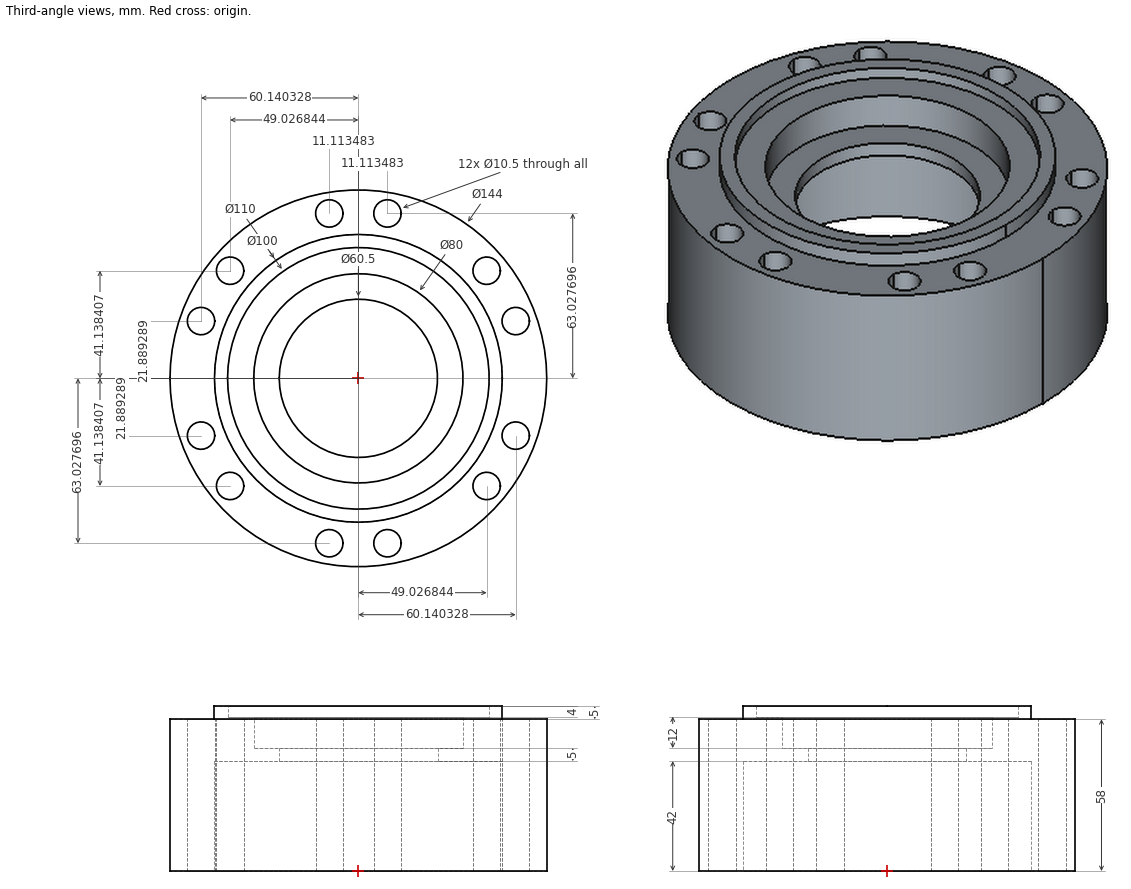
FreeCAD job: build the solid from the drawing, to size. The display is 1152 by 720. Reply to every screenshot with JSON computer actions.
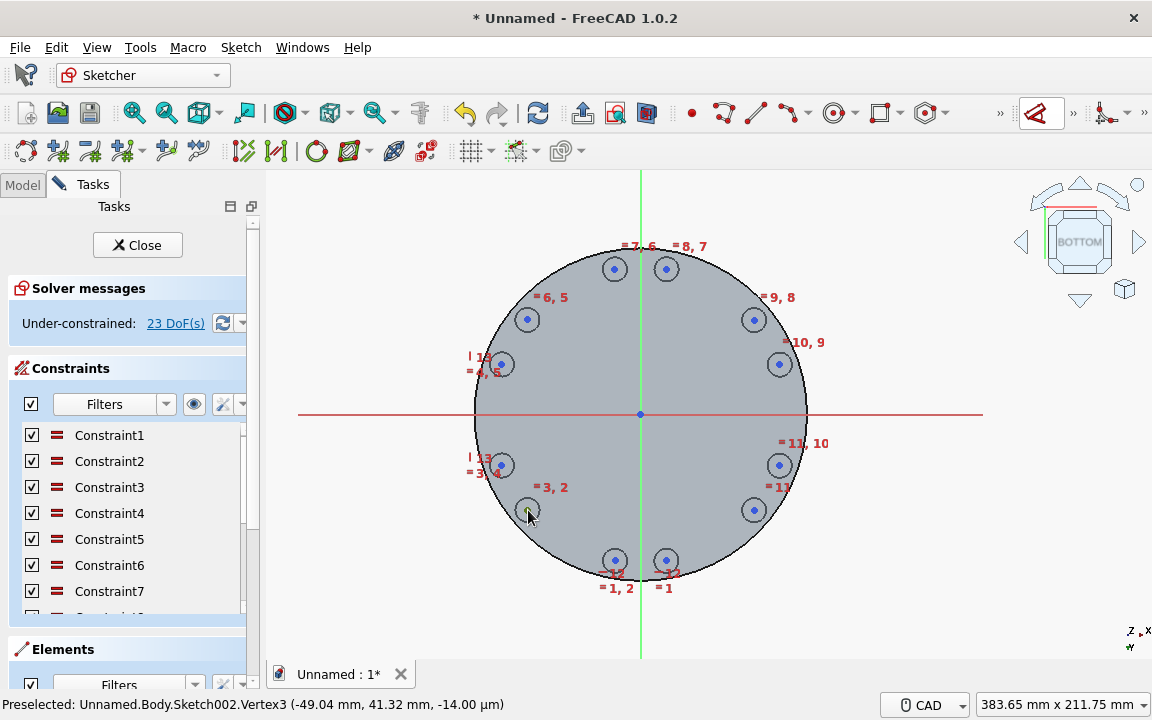
{"action": "left_click", "coordinate": [527, 320]}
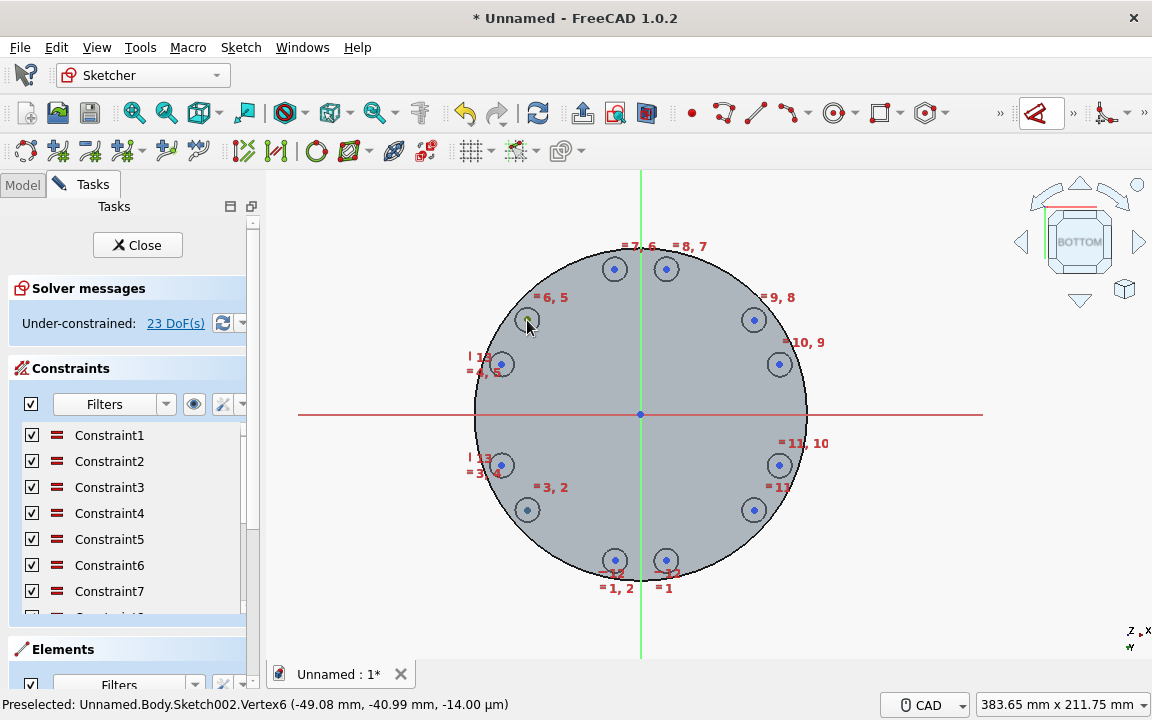
{"action": "key", "text": "v"}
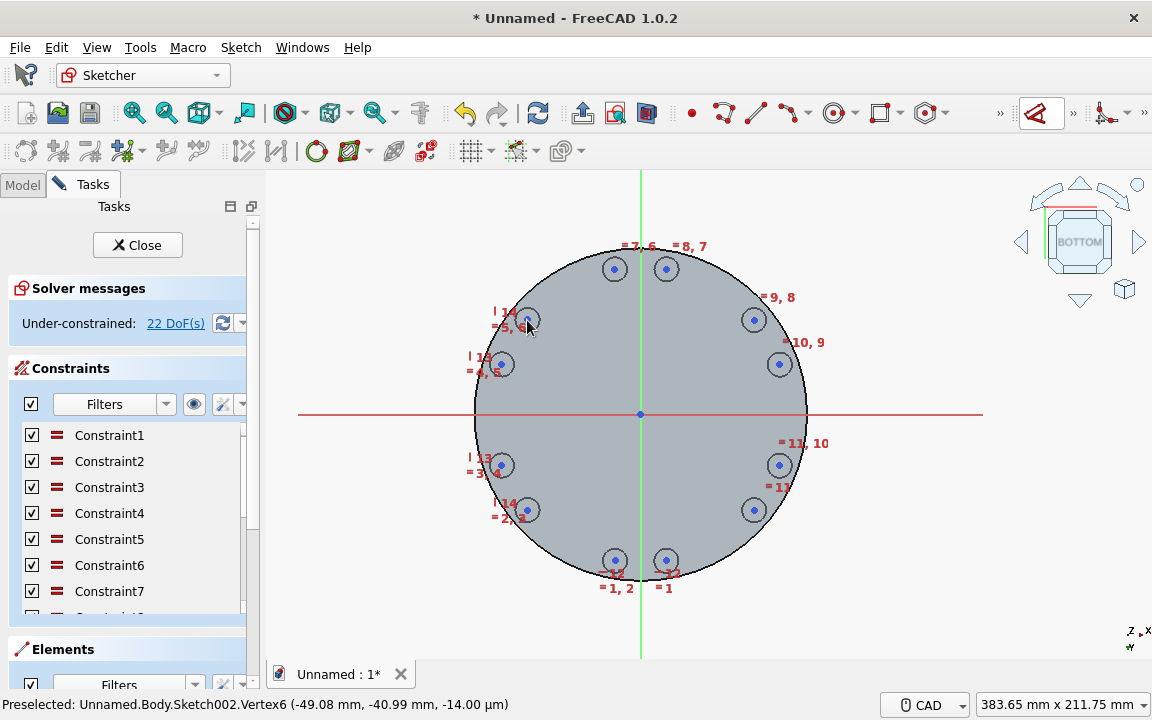
{"action": "left_click", "coordinate": [615, 561]}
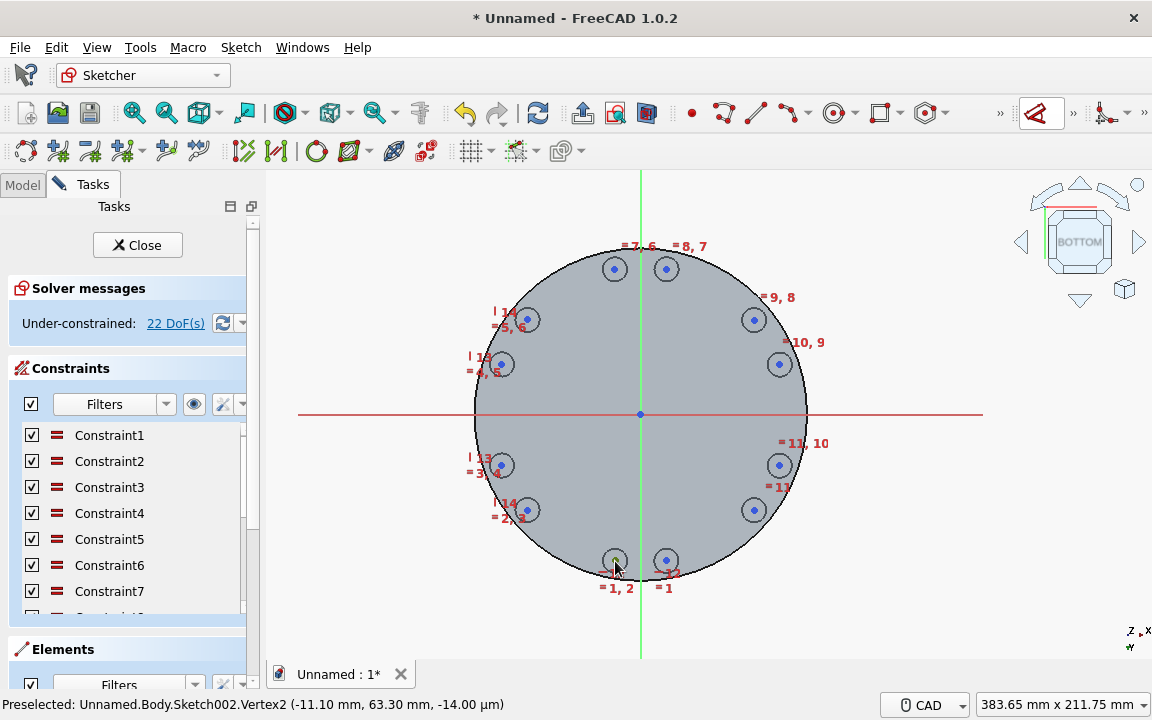
{"action": "left_click", "coordinate": [615, 269]}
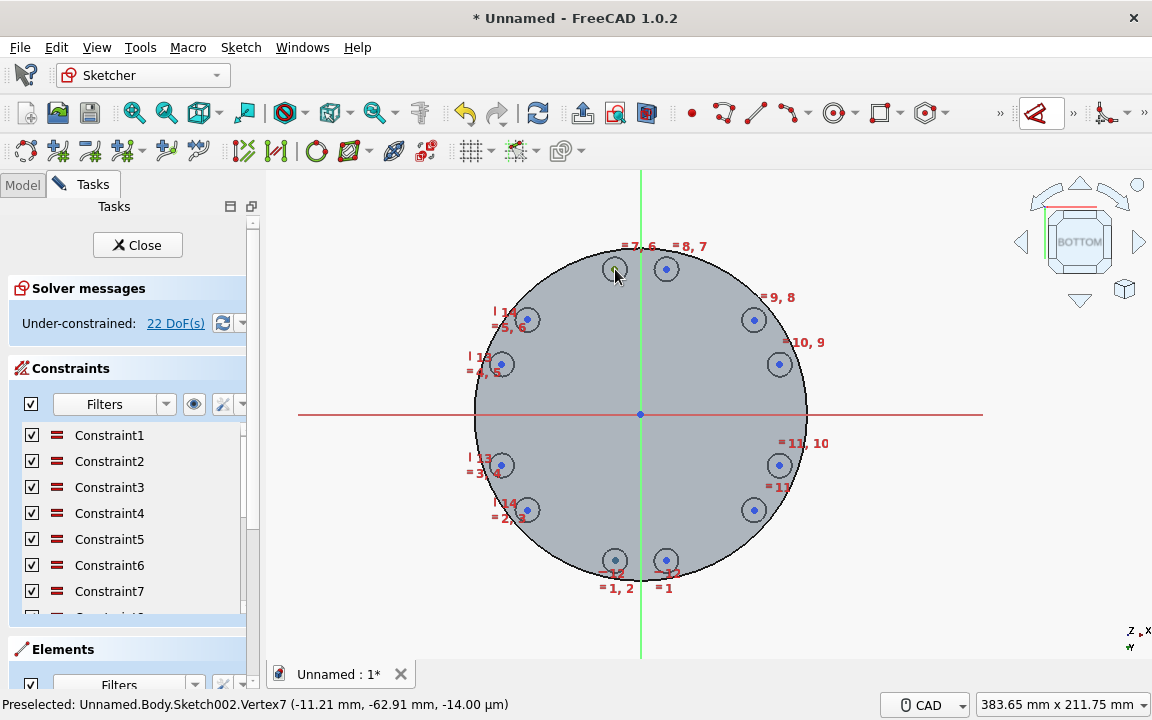
{"action": "key", "text": "v"}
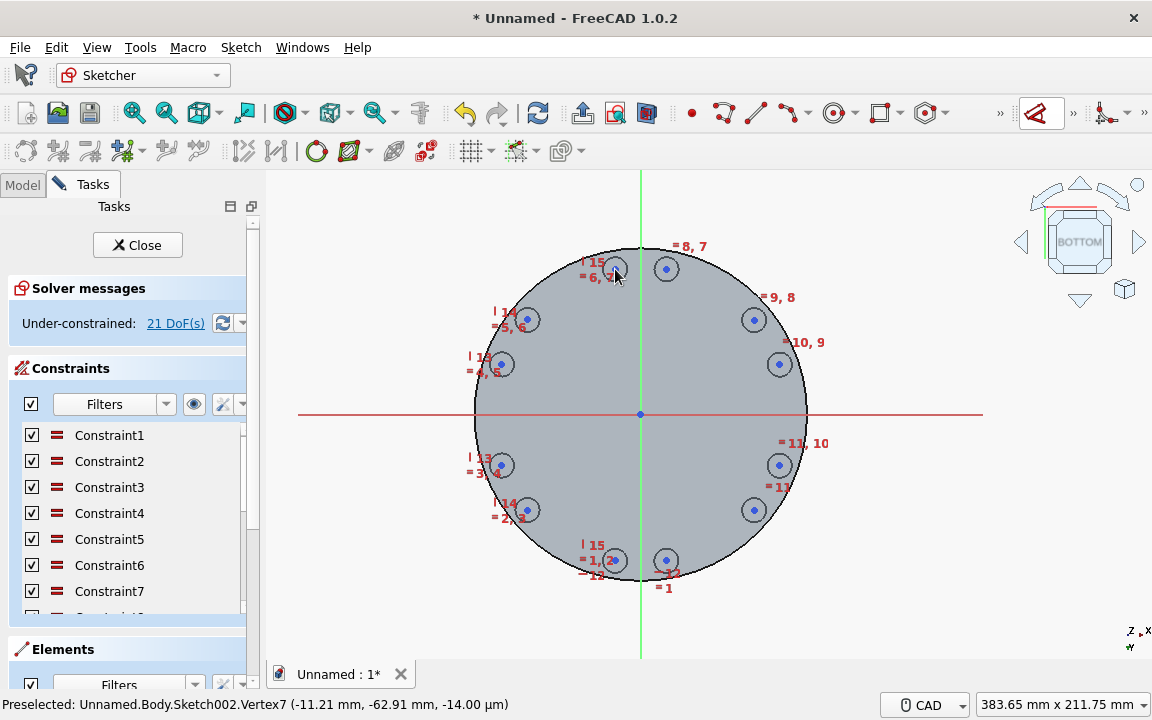
{"action": "left_click", "coordinate": [666, 561]}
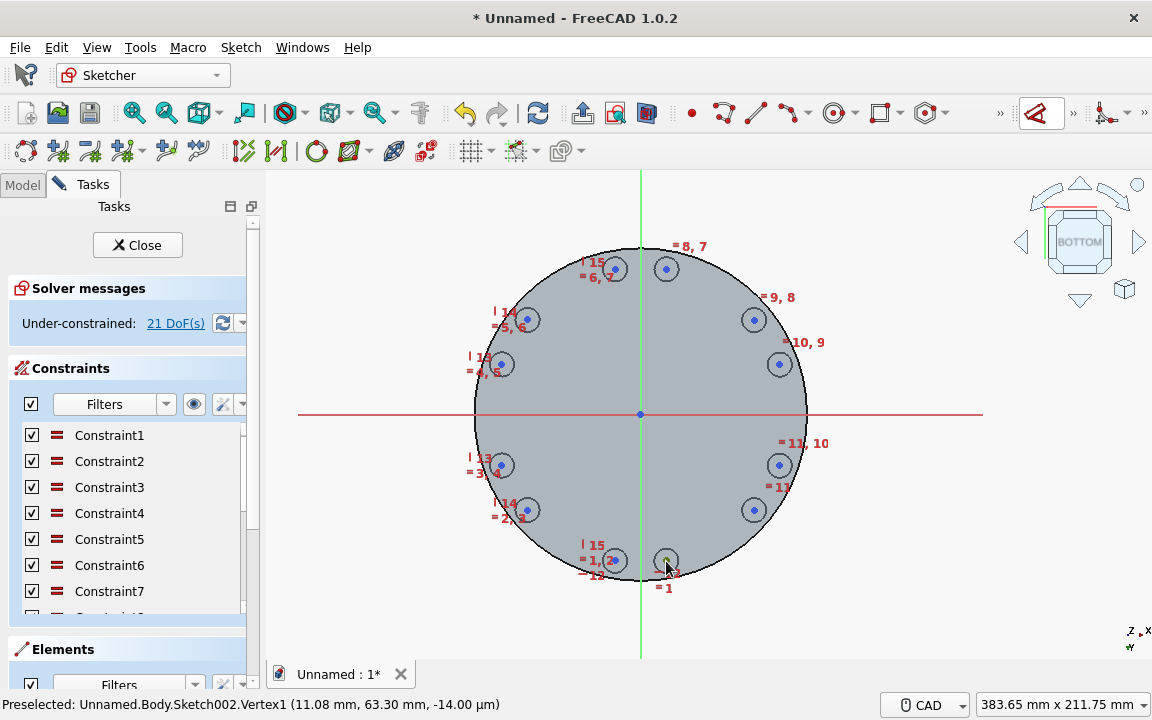
{"action": "left_click", "coordinate": [667, 269]}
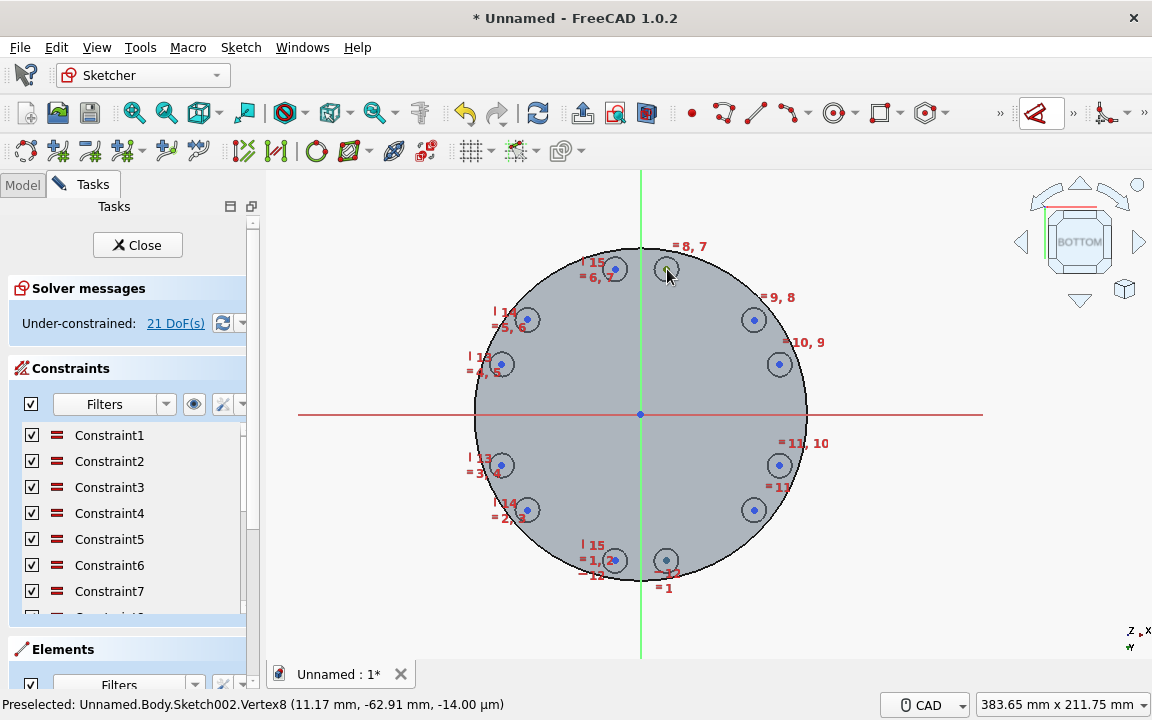
{"action": "key", "text": "v"}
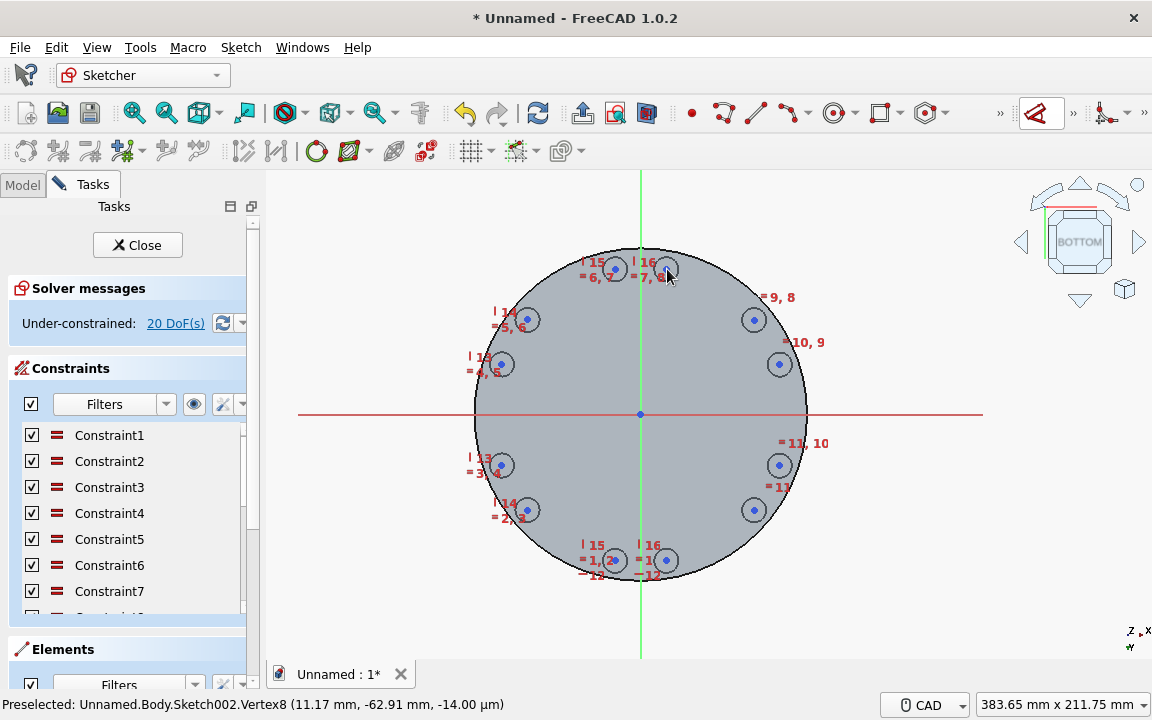
{"action": "left_click", "coordinate": [615, 269]}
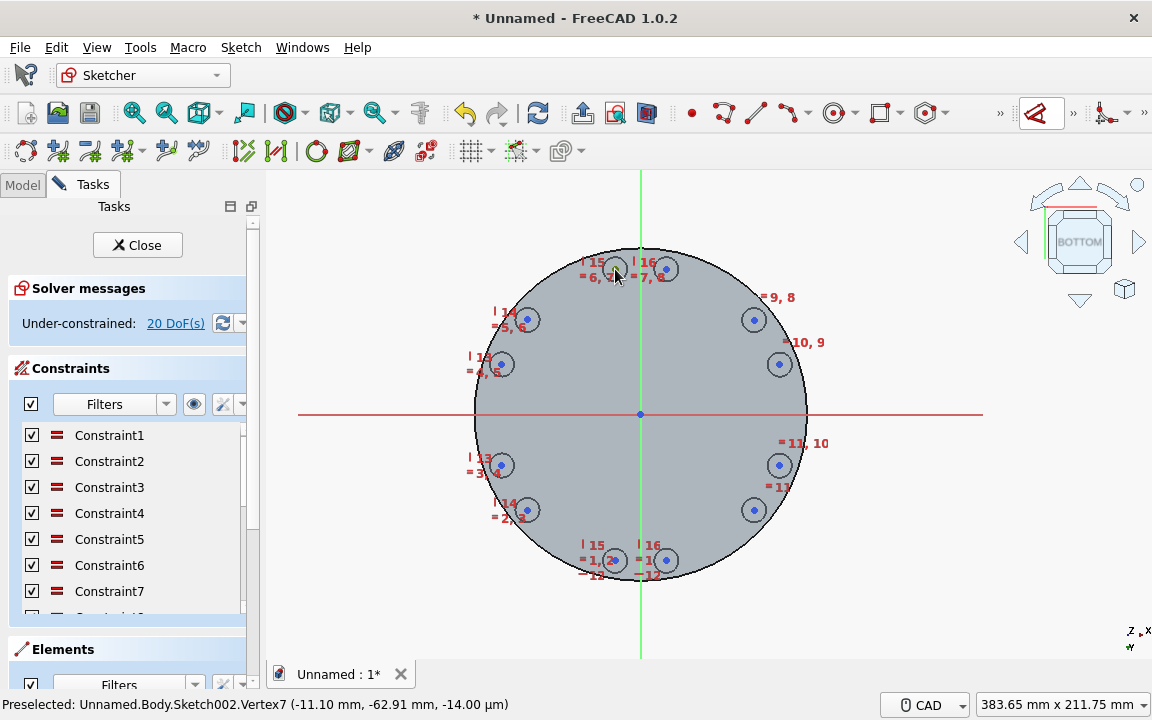
{"action": "left_click", "coordinate": [666, 269]}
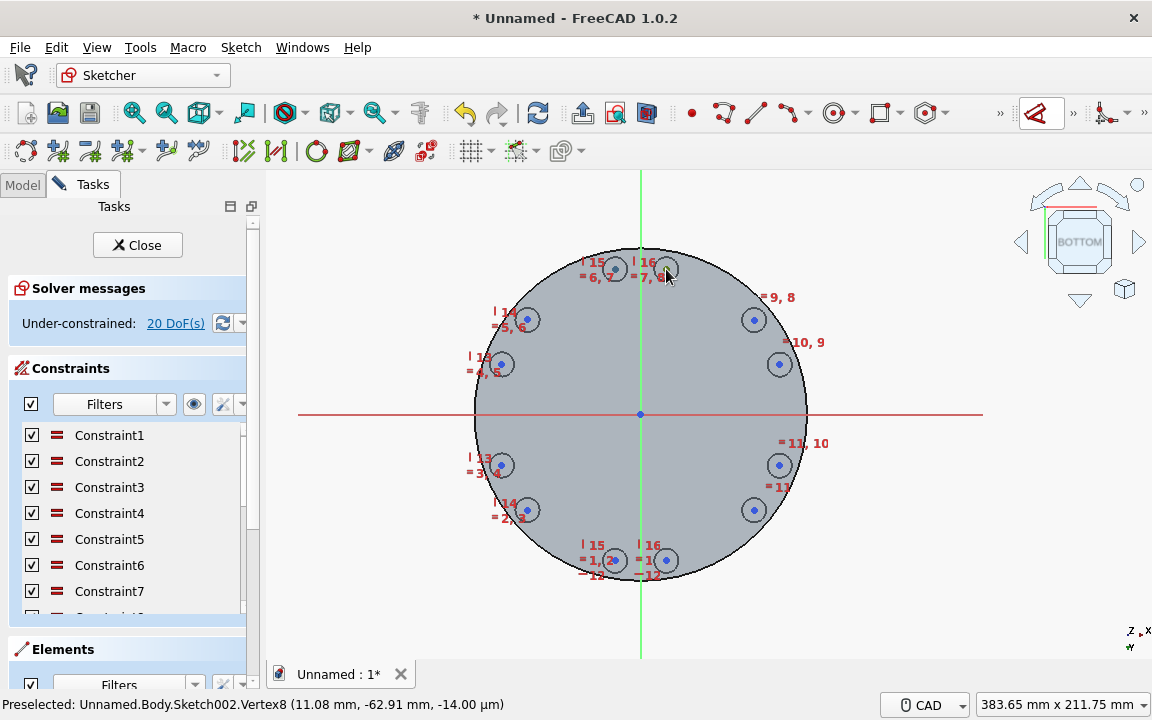
{"action": "key", "text": "h"}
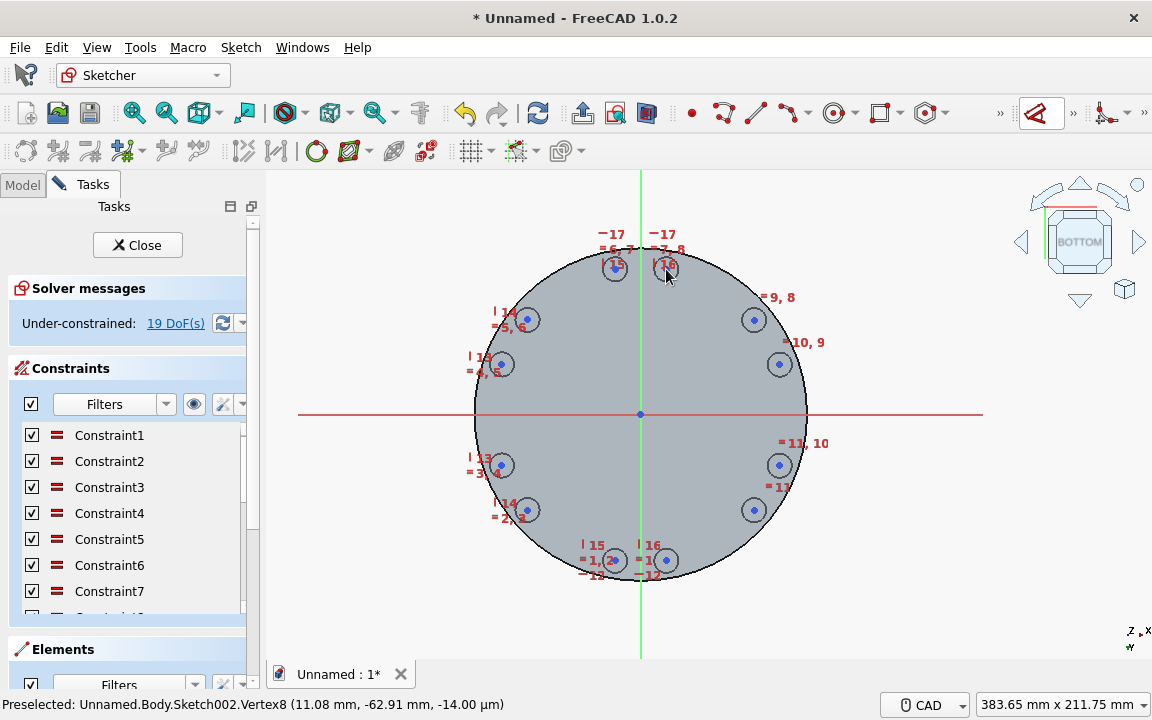
{"action": "left_click", "coordinate": [528, 320]}